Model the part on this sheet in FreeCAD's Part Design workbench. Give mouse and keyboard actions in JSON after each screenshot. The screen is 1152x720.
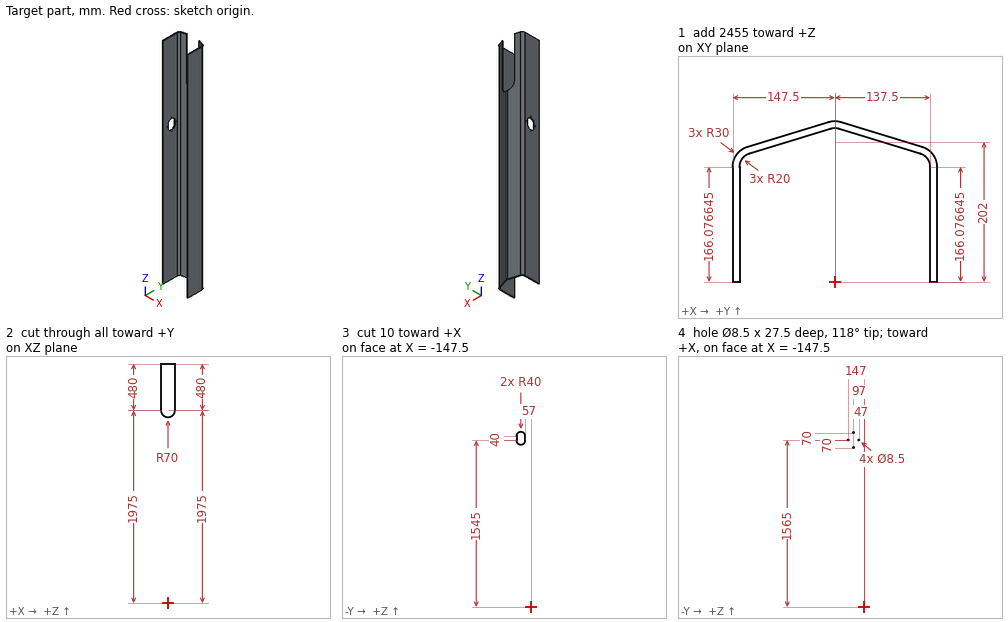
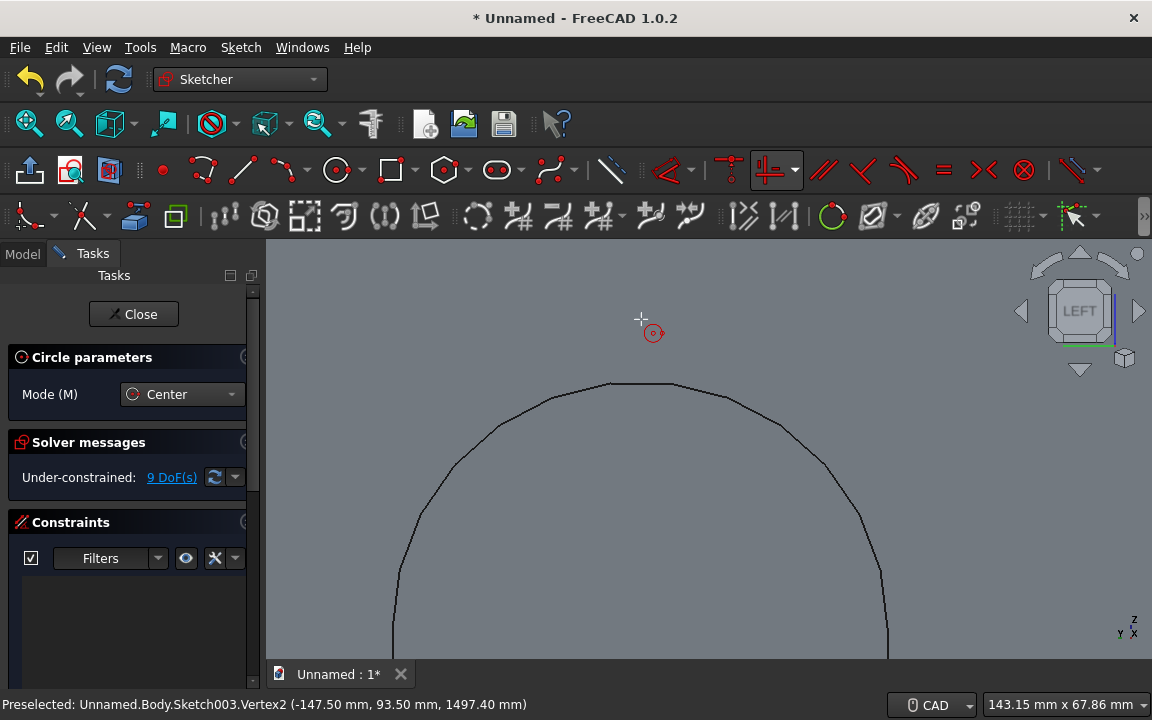
{"action": "left_click", "coordinate": [640, 320]}
{"action": "left_click", "coordinate": [659, 301]}
{"action": "key", "text": "Escape"}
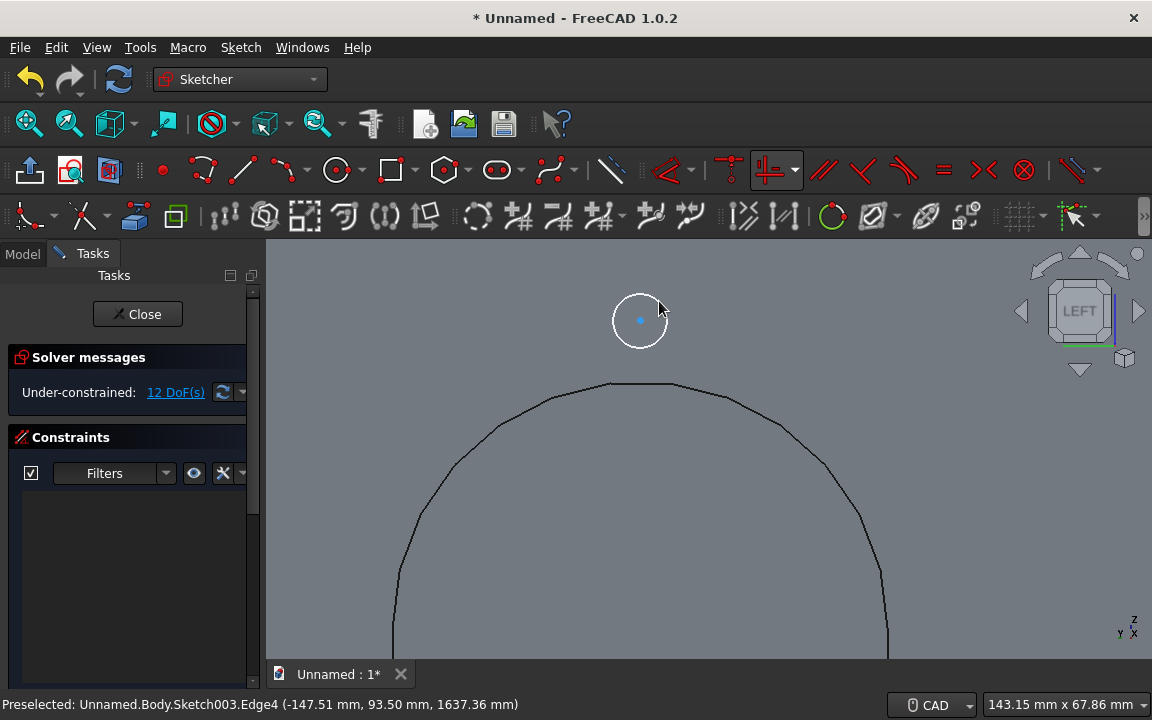
{"action": "scroll", "coordinate": [641, 318], "scroll_direction": "down", "scroll_amount": 6}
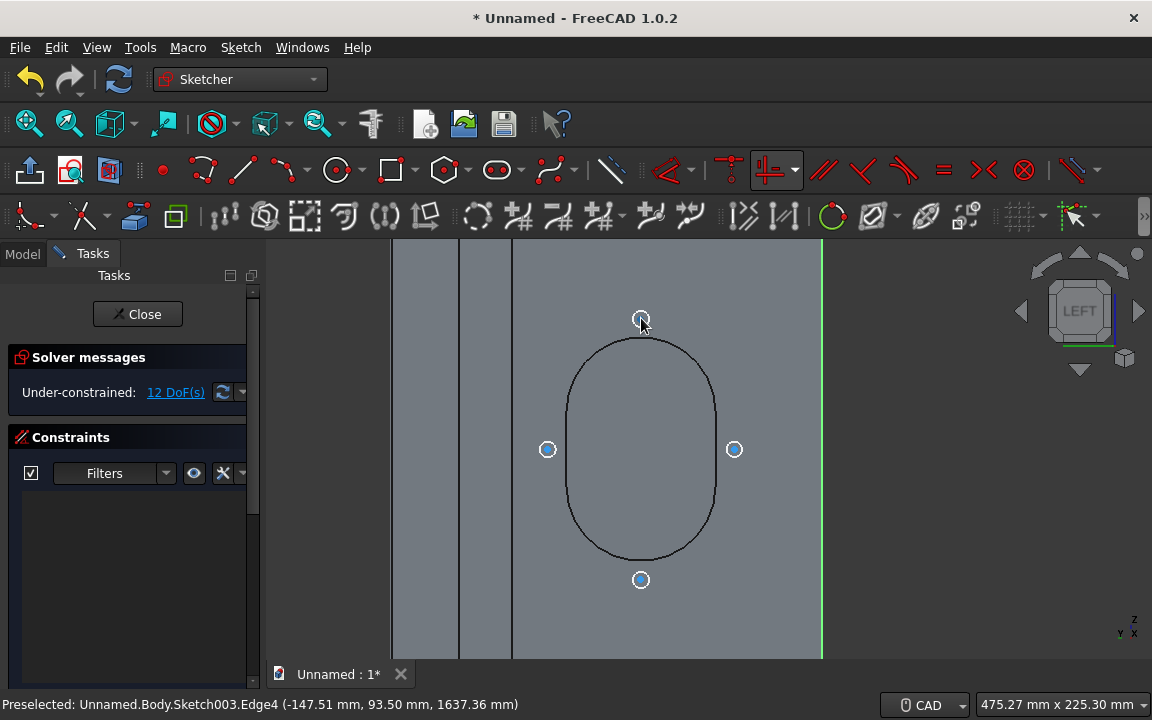
{"action": "scroll", "coordinate": [553, 444], "scroll_direction": "up", "scroll_amount": 3}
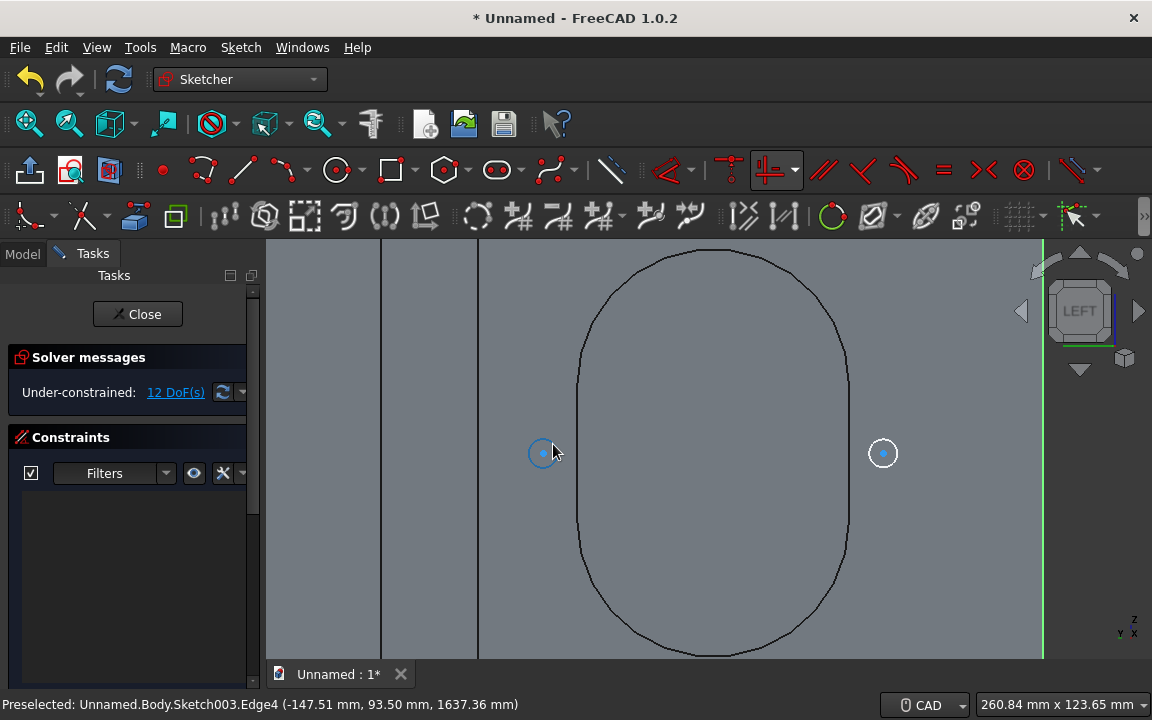
{"action": "left_click", "coordinate": [553, 443]}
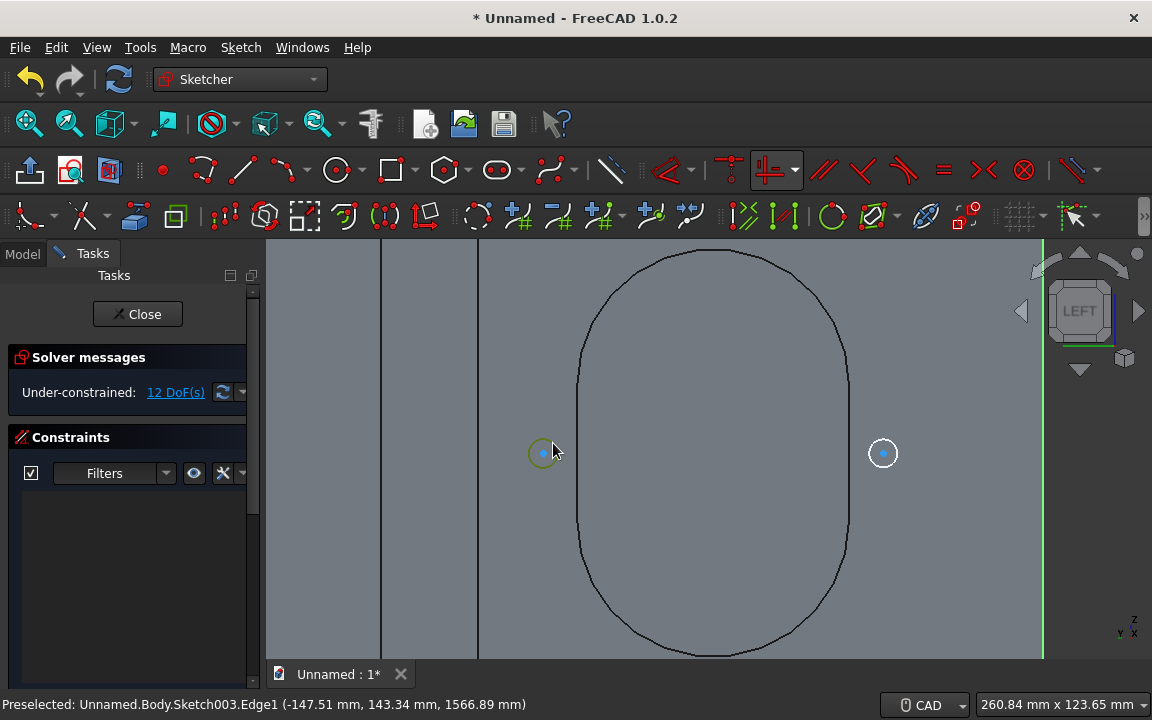
{"action": "left_click", "coordinate": [893, 443]}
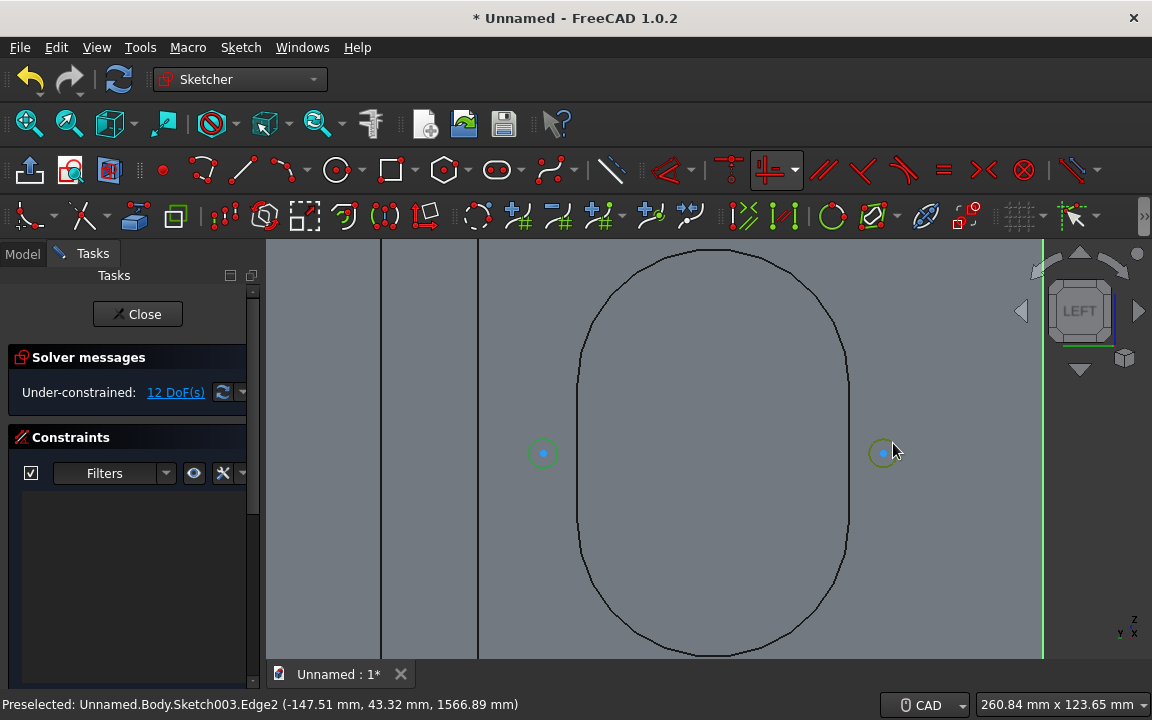
{"action": "scroll", "coordinate": [552, 444], "scroll_direction": "down", "scroll_amount": 3}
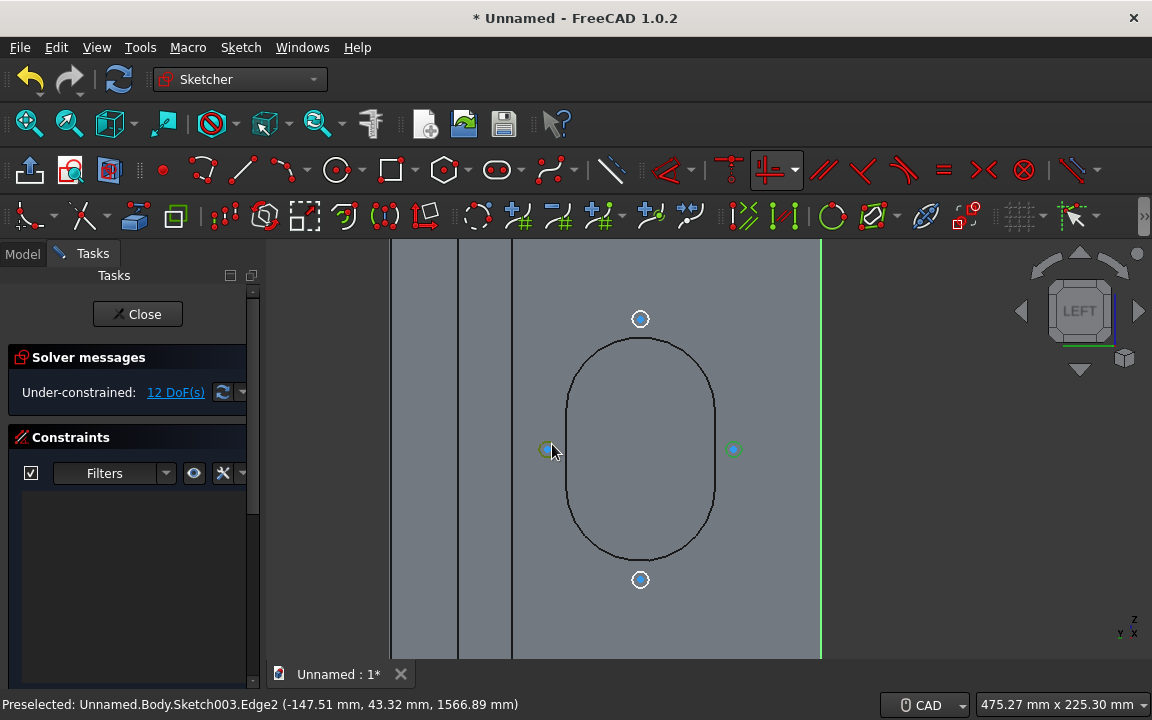
{"action": "scroll", "coordinate": [646, 574], "scroll_direction": "up", "scroll_amount": 3}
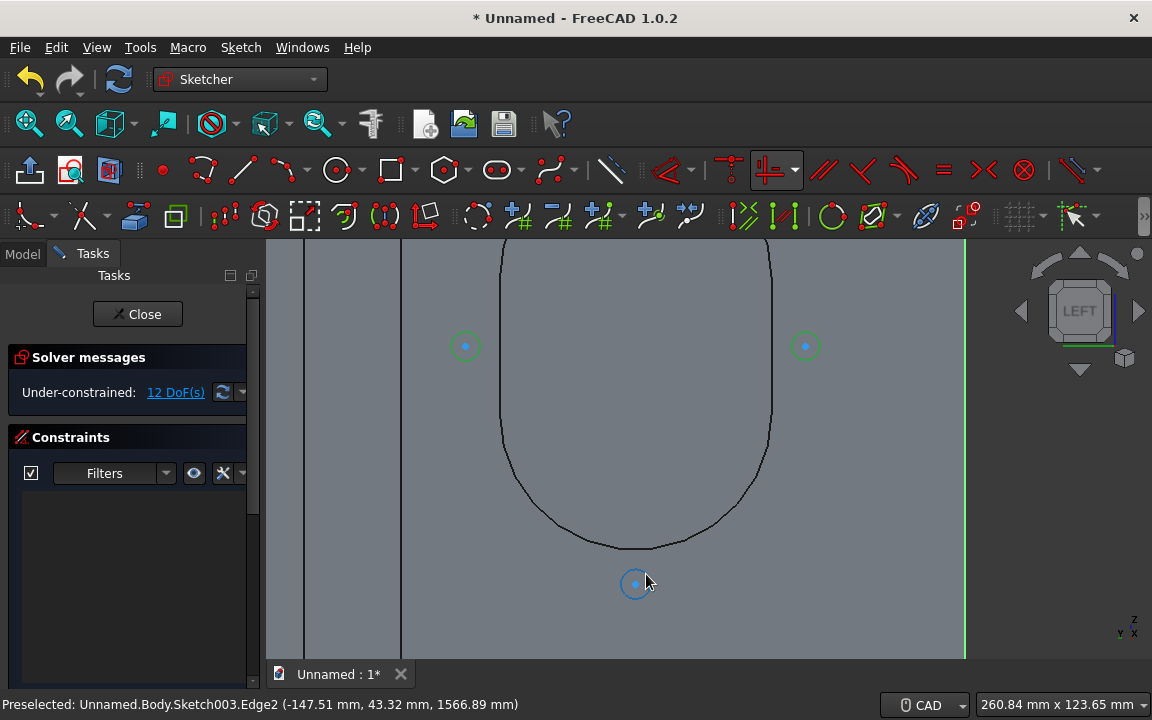
{"action": "left_click", "coordinate": [646, 574]}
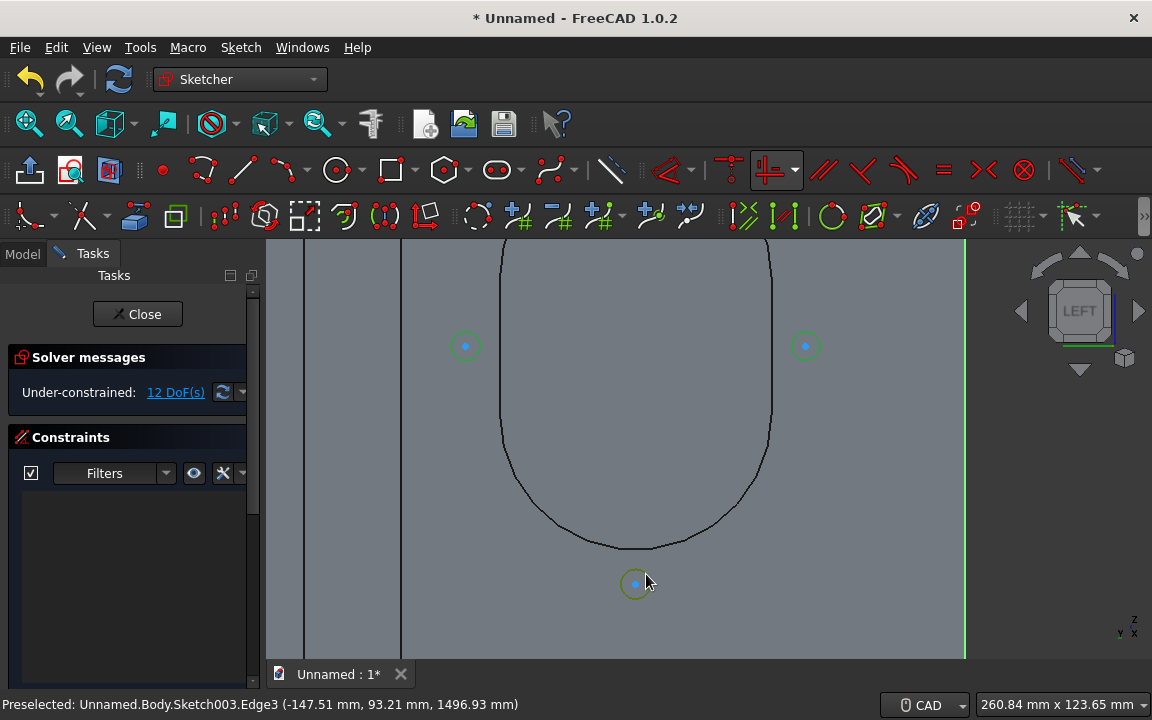
{"action": "scroll", "coordinate": [646, 574], "scroll_direction": "down", "scroll_amount": 3}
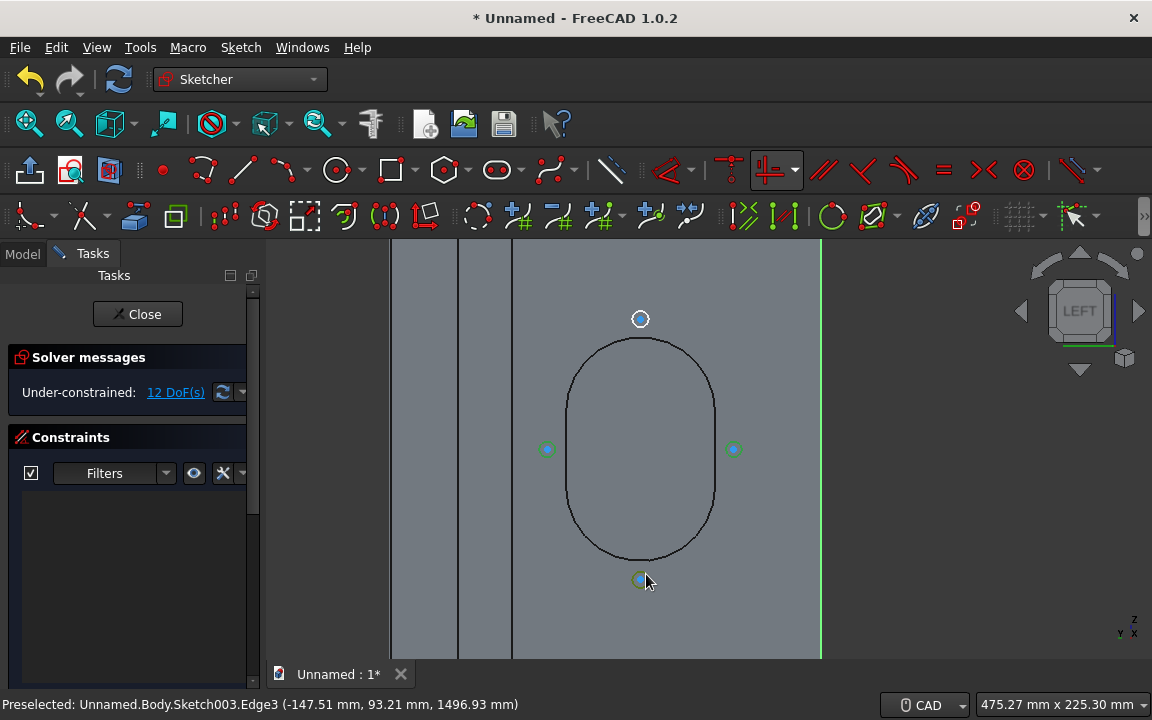
{"action": "scroll", "coordinate": [646, 313], "scroll_direction": "up", "scroll_amount": 3}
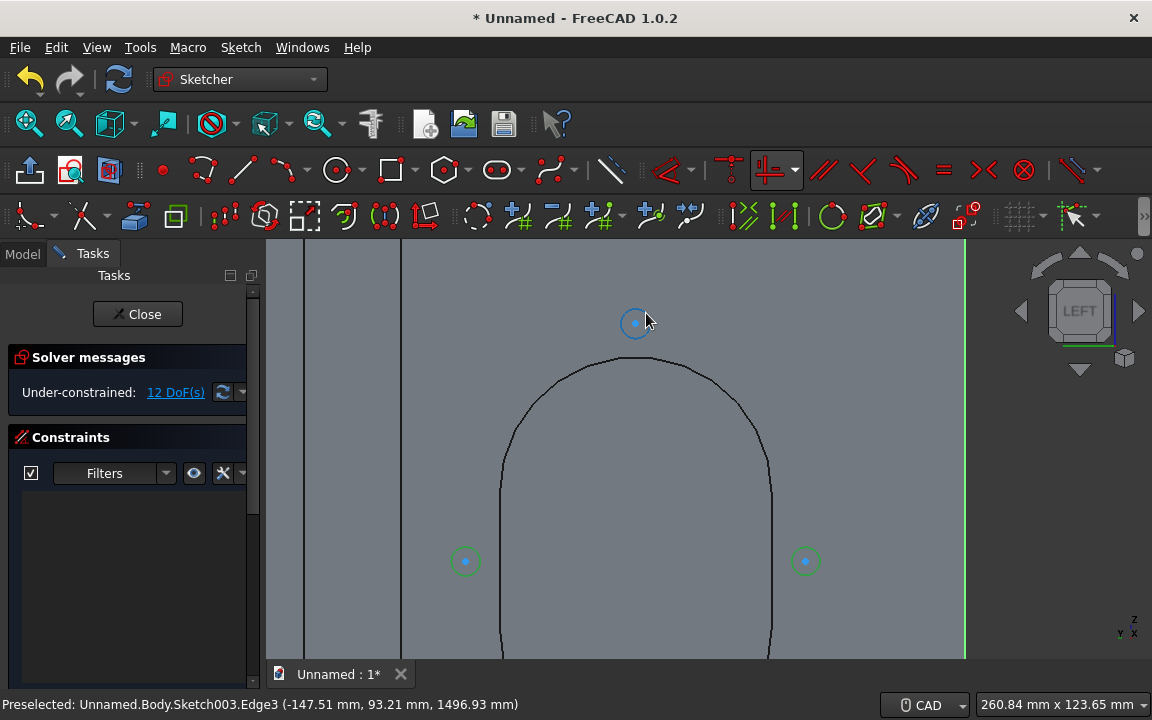
{"action": "left_click", "coordinate": [646, 313]}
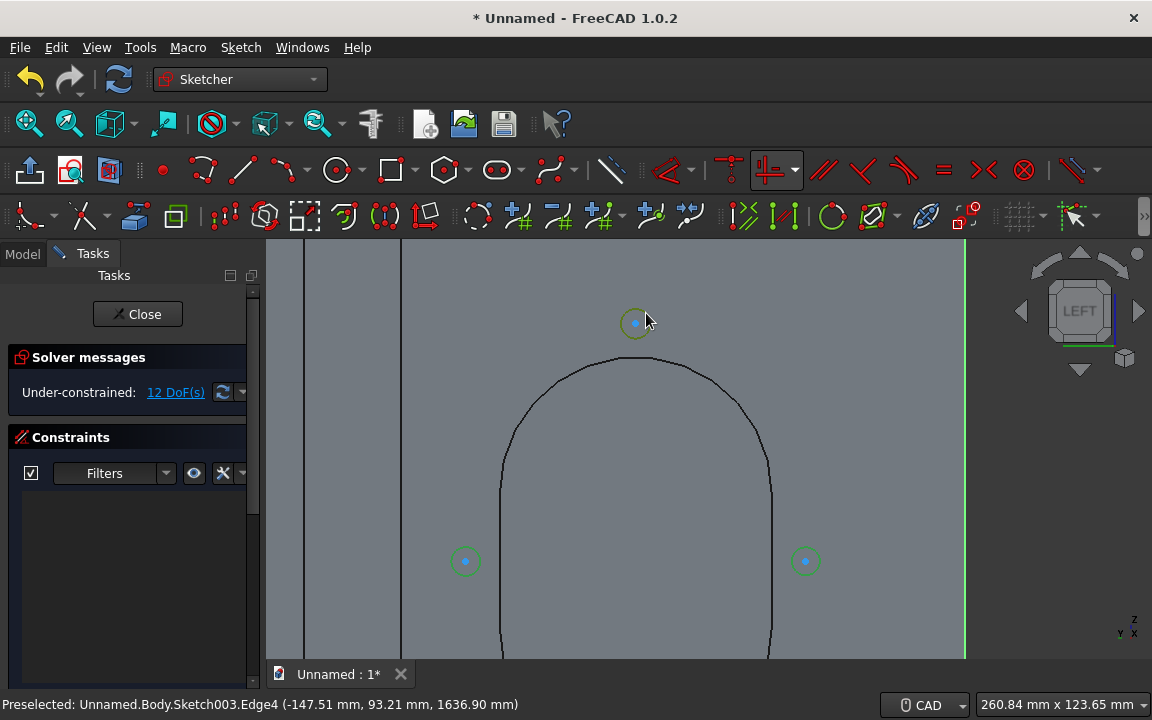
{"action": "left_click", "coordinate": [944, 170]}